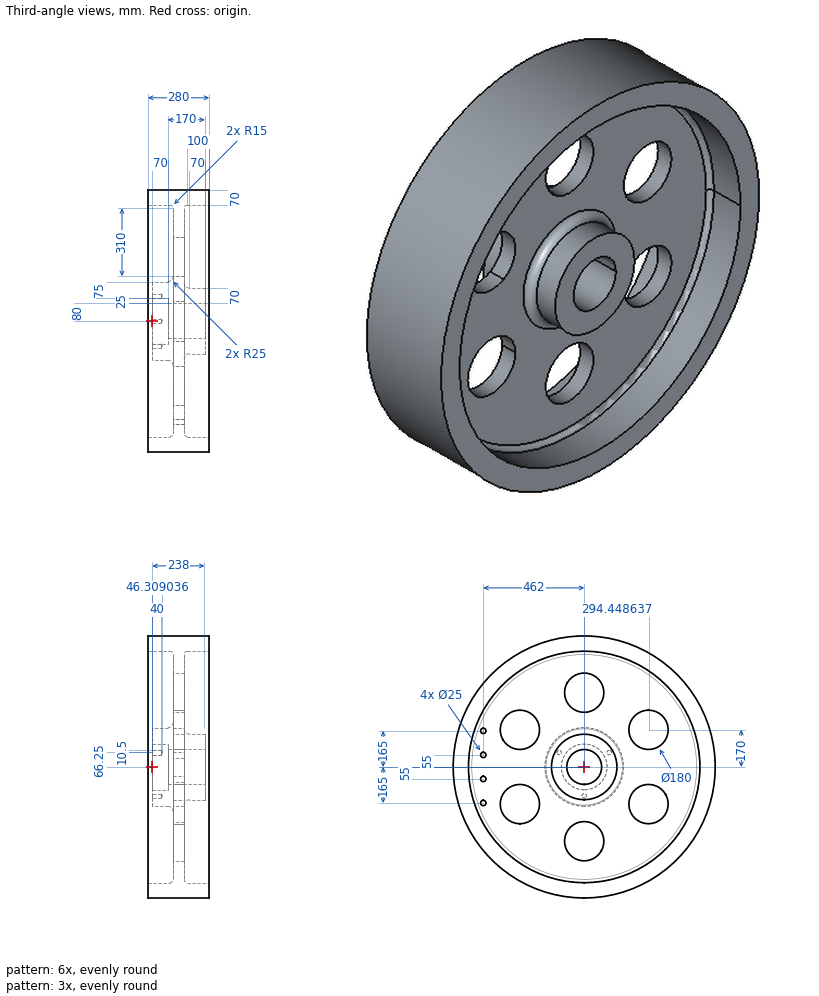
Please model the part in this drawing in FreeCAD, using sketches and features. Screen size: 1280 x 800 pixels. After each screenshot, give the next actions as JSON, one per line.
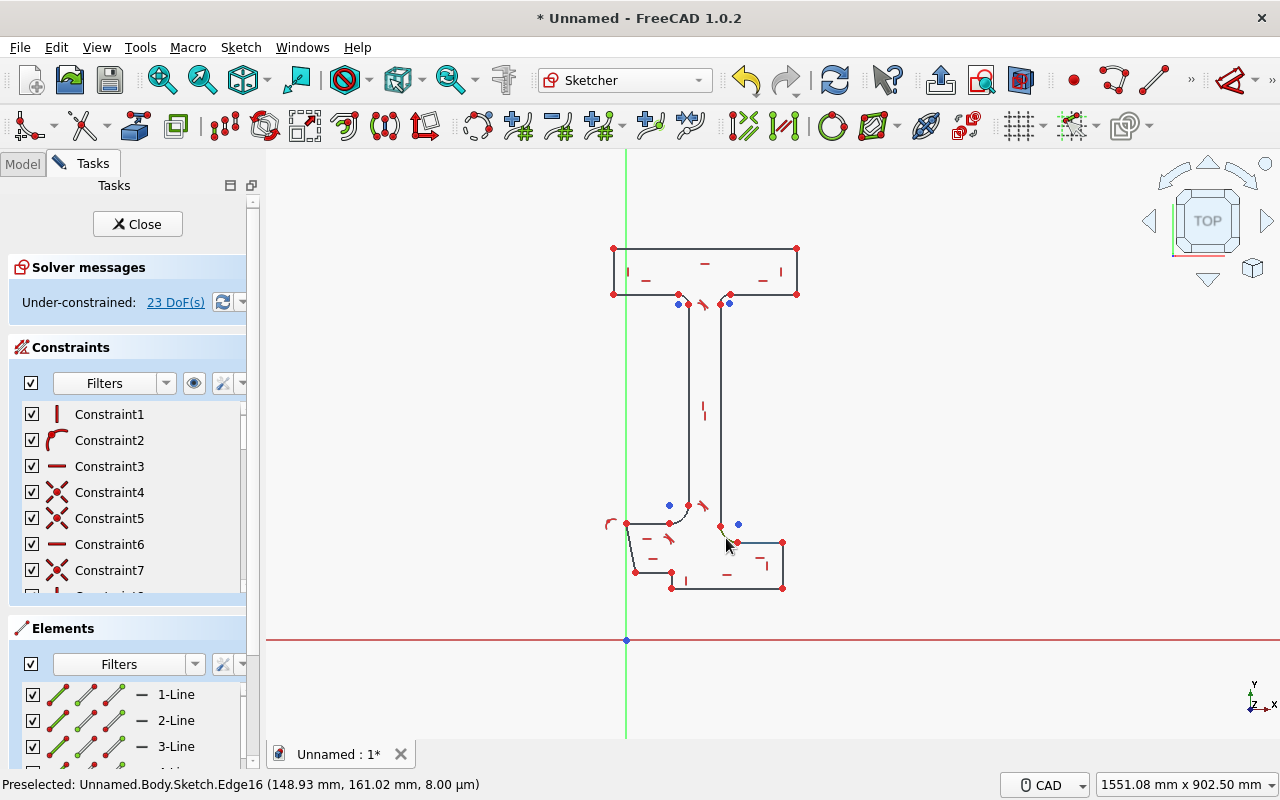
{"action": "key", "text": "t"}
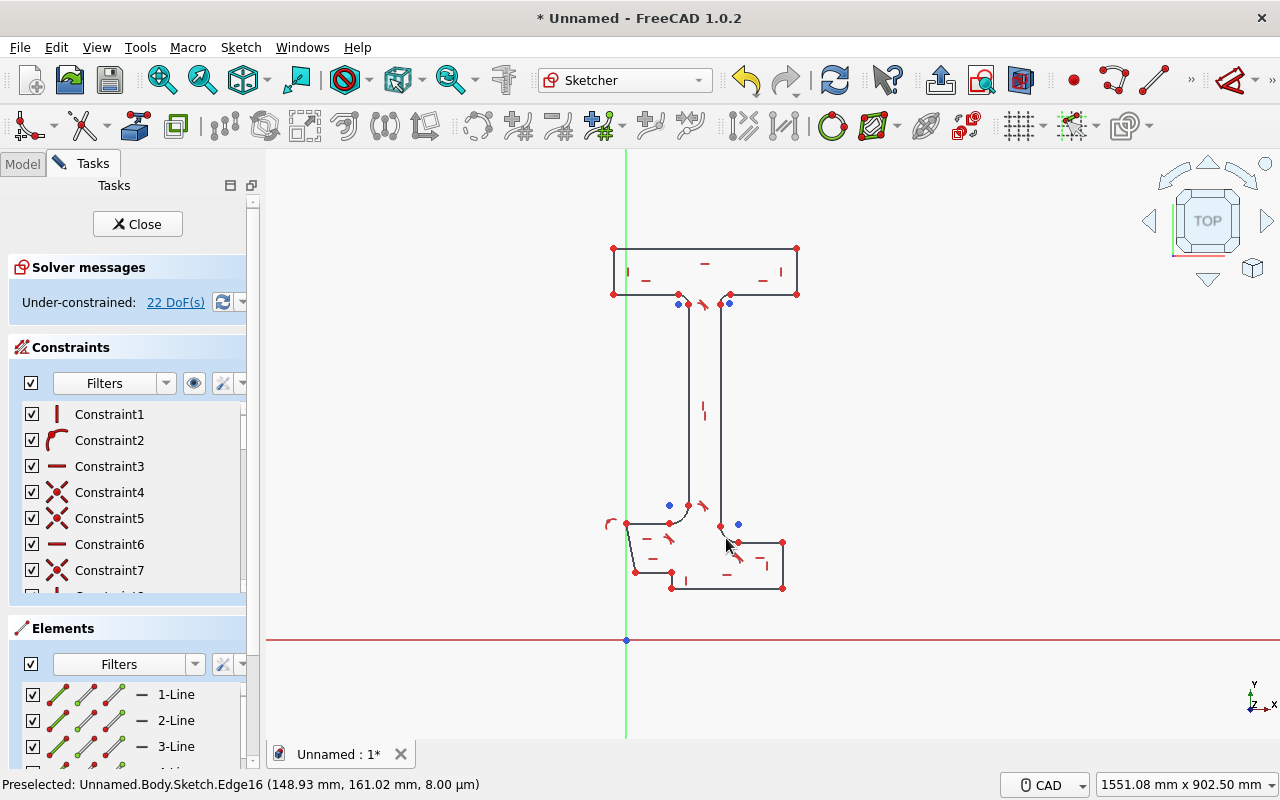
{"action": "left_click", "coordinate": [721, 460]}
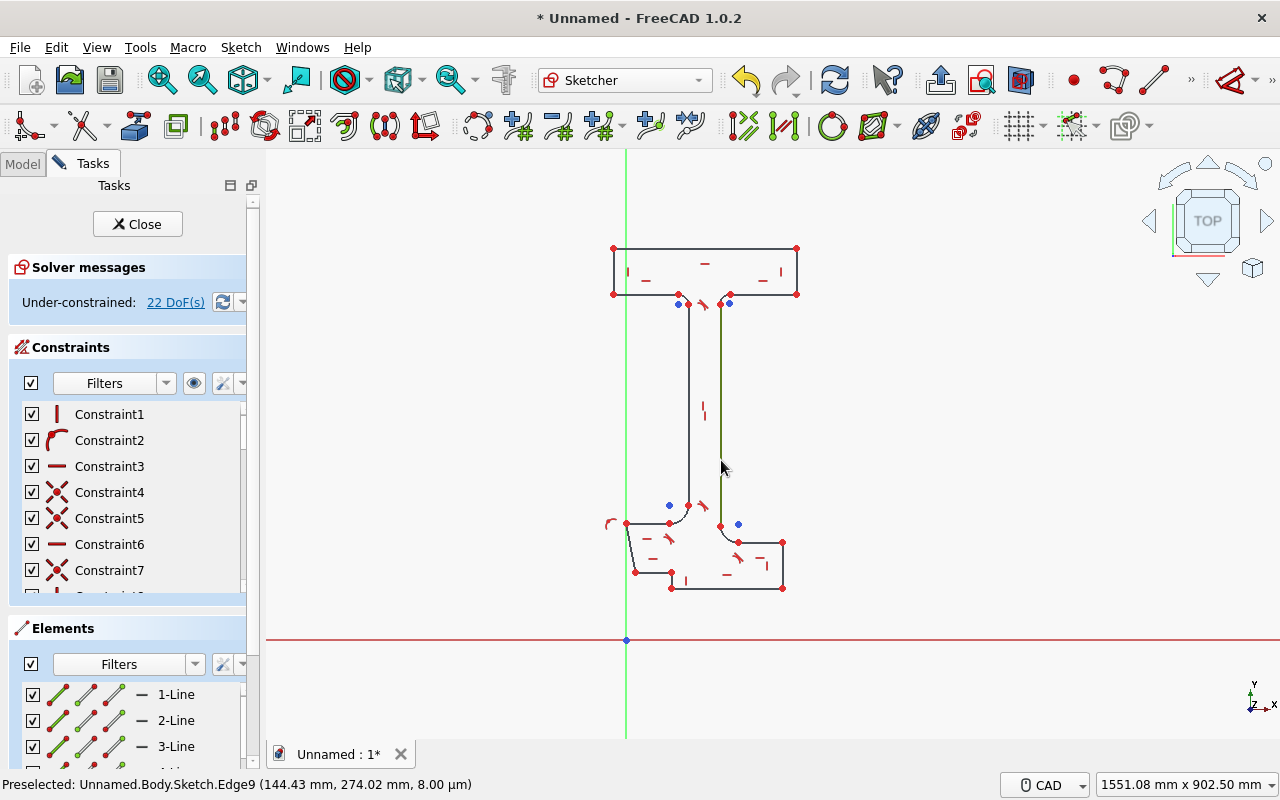
{"action": "left_click", "coordinate": [726, 538]}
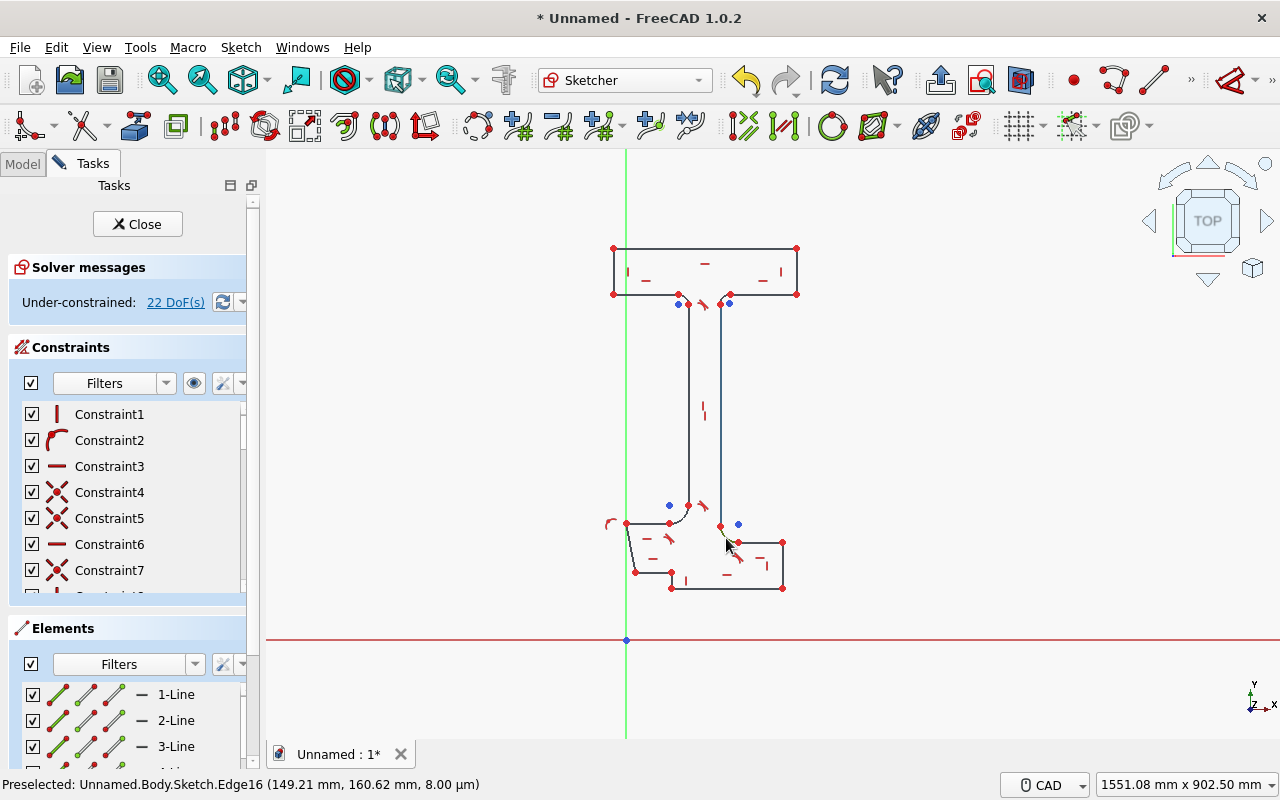
{"action": "key", "text": "t"}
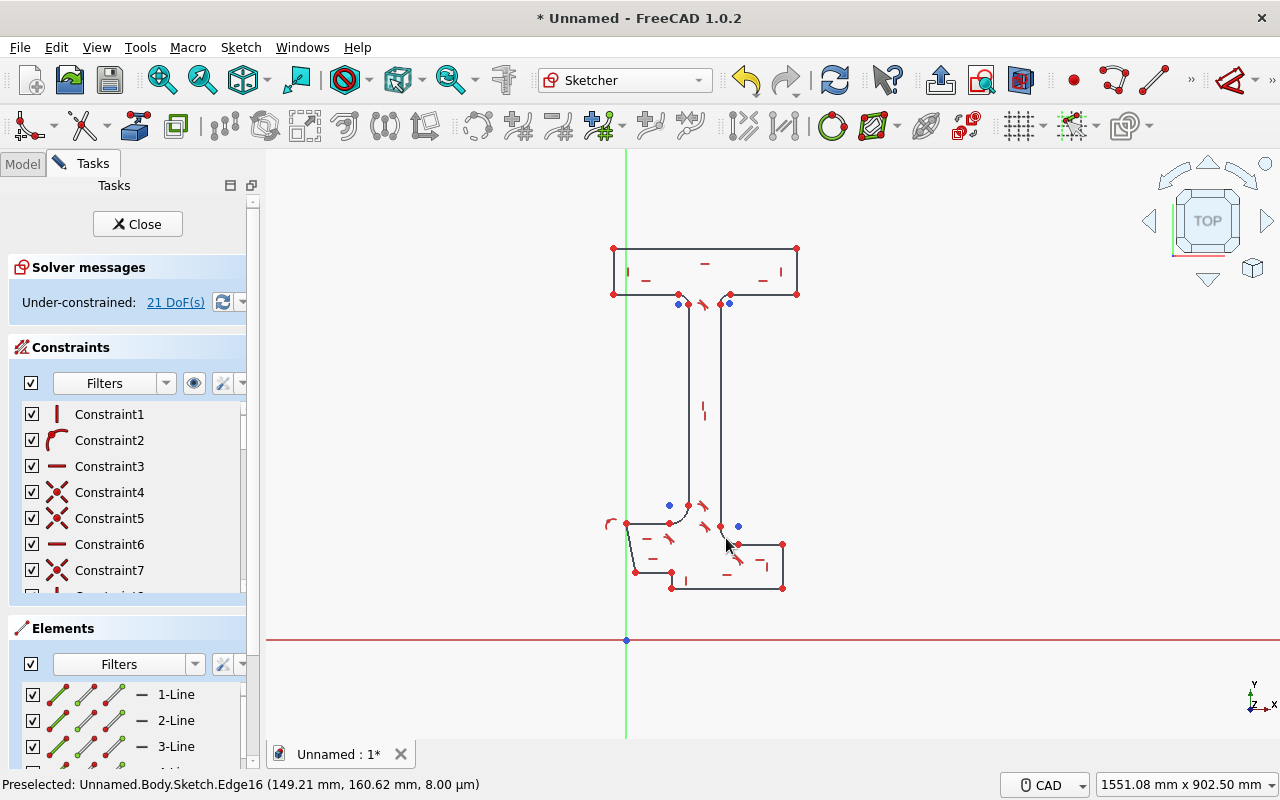
{"action": "left_click", "coordinate": [721, 460]}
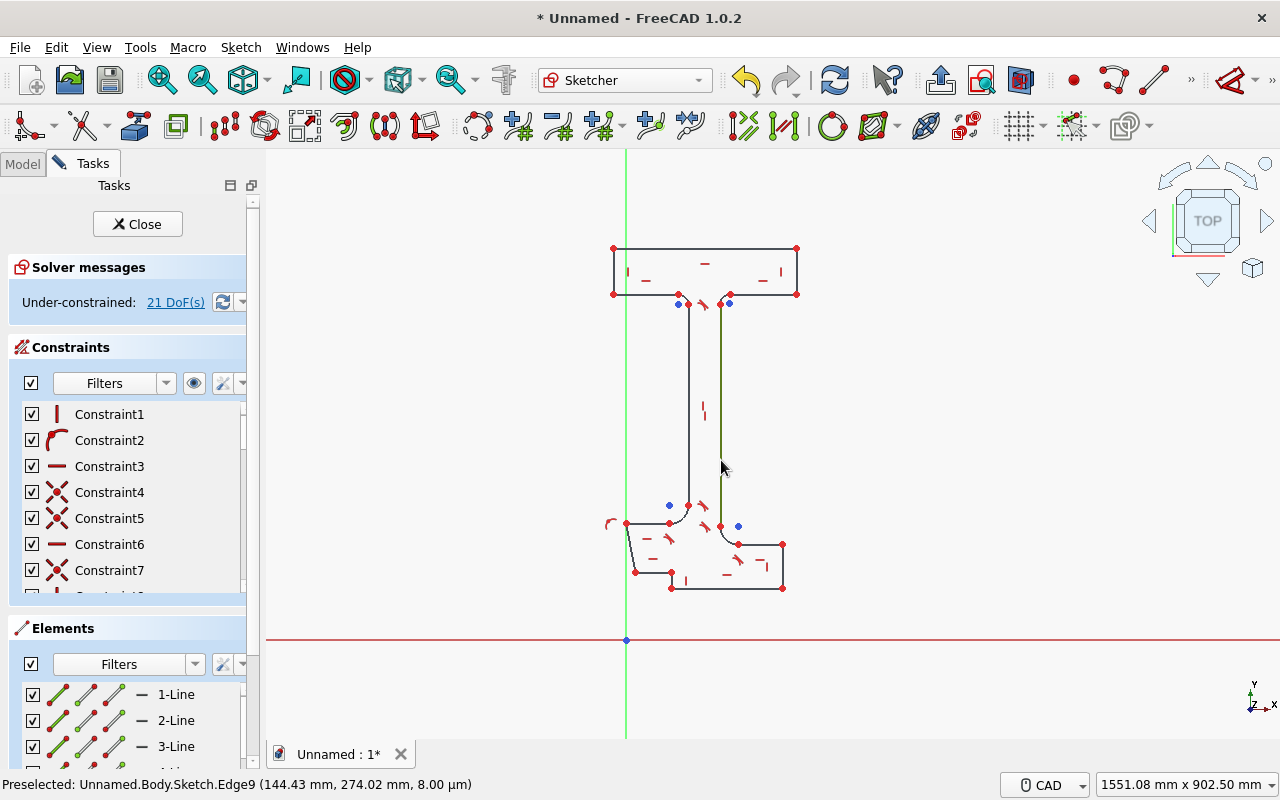
{"action": "scroll", "coordinate": [723, 297], "scroll_direction": "up", "scroll_amount": 3}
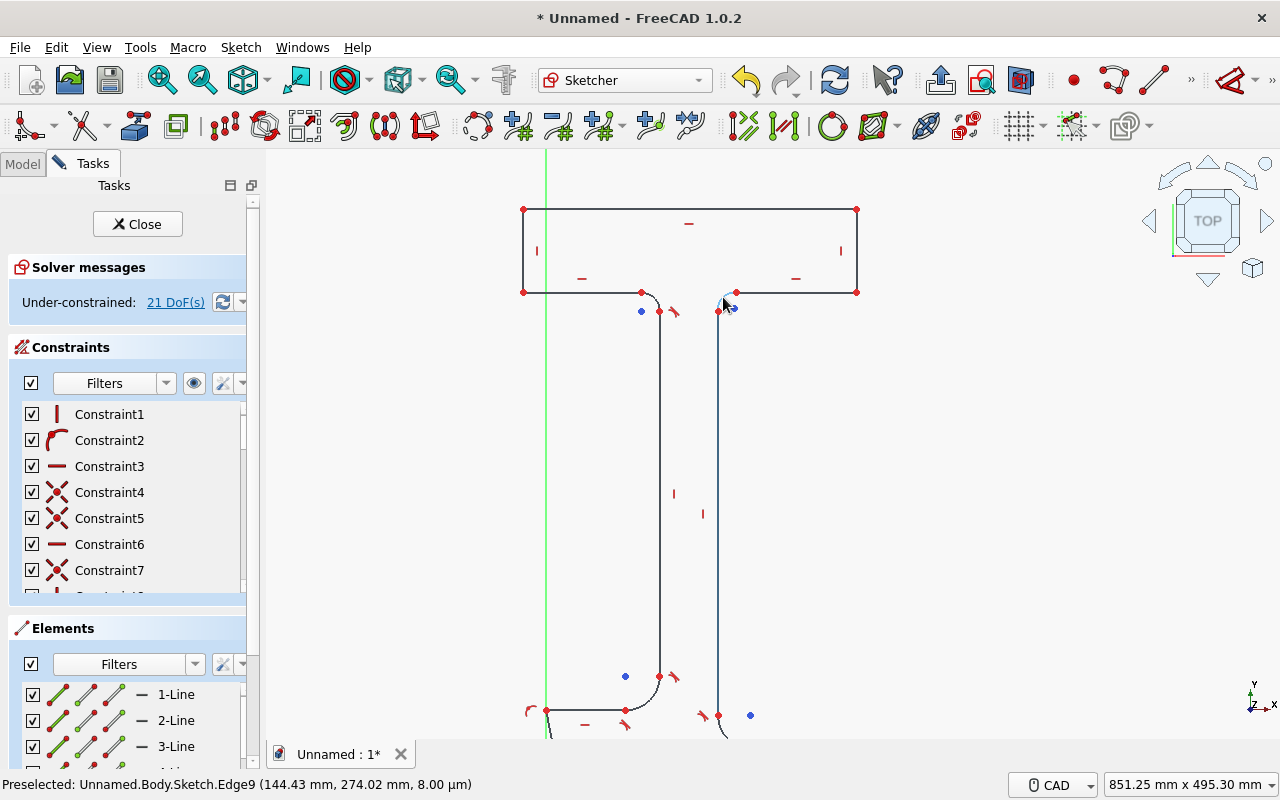
{"action": "left_click", "coordinate": [723, 297]}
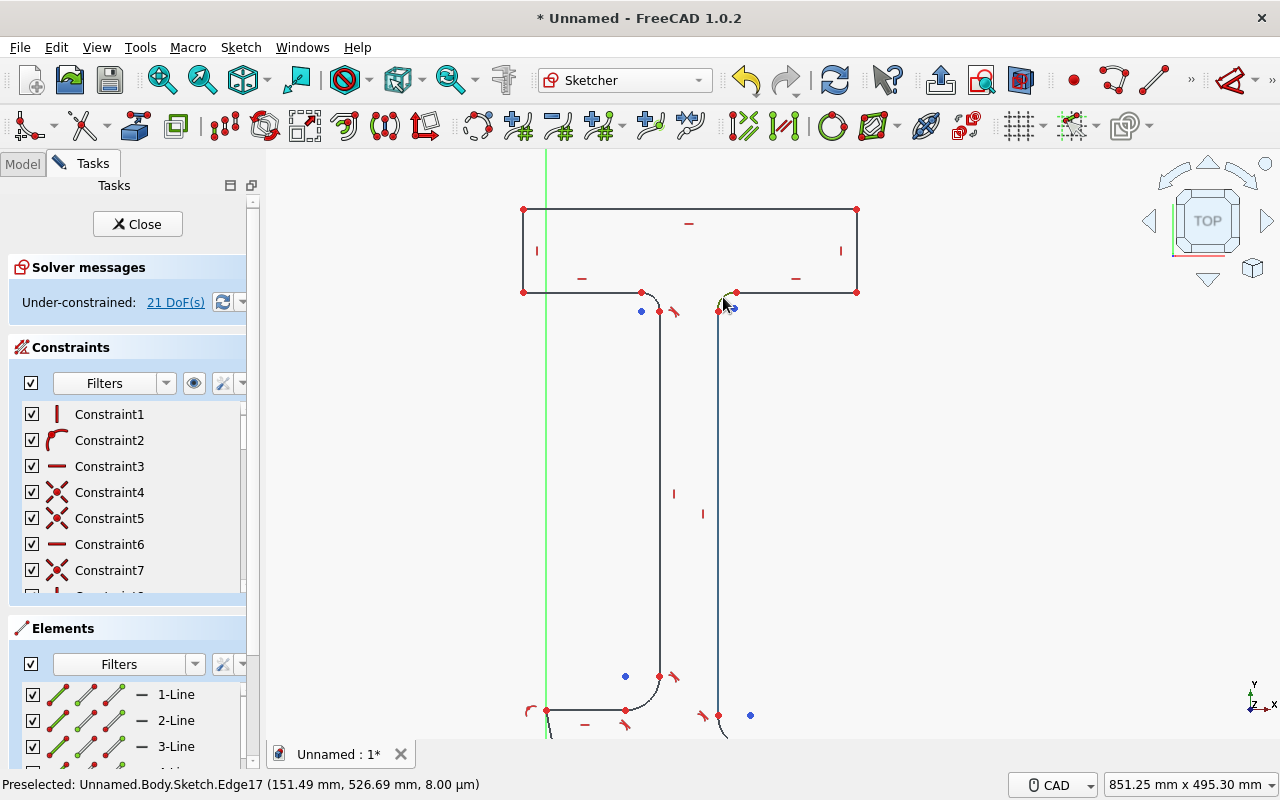
{"action": "key", "text": "t"}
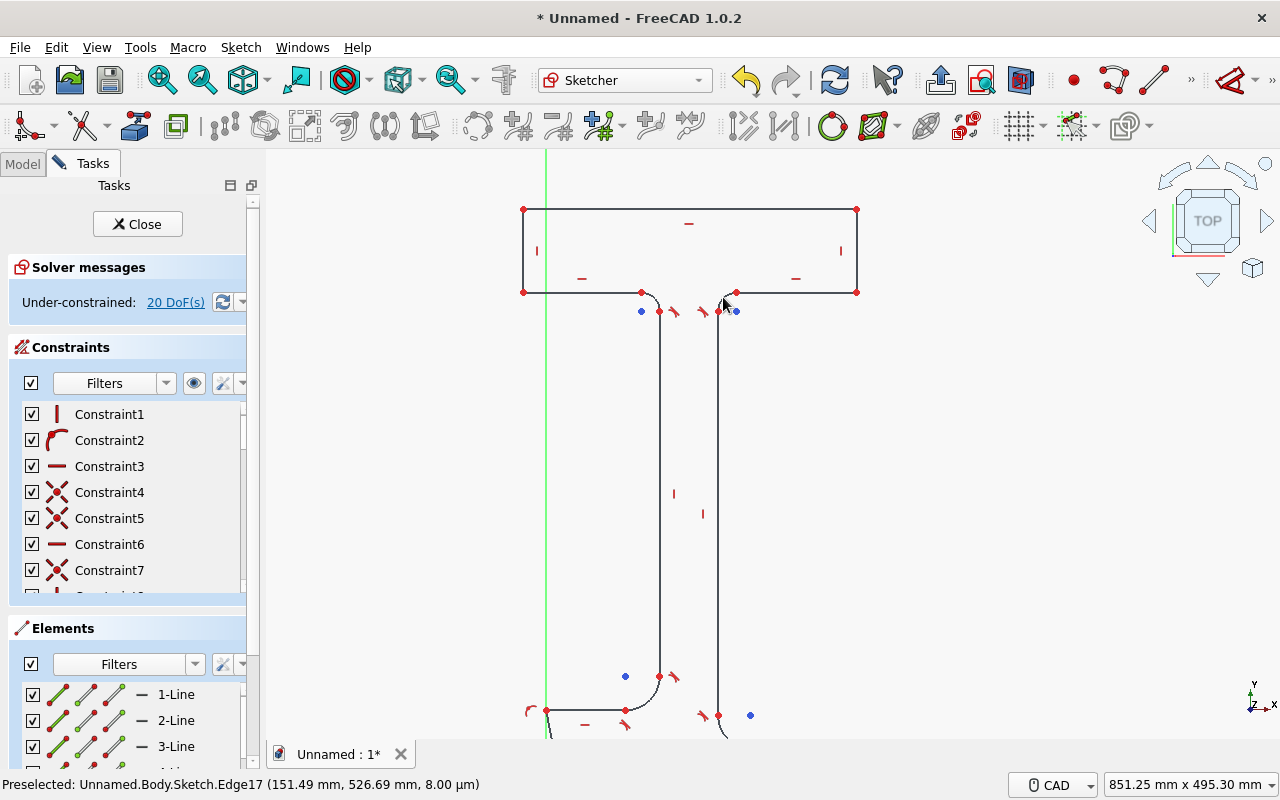
{"action": "left_click", "coordinate": [772, 293]}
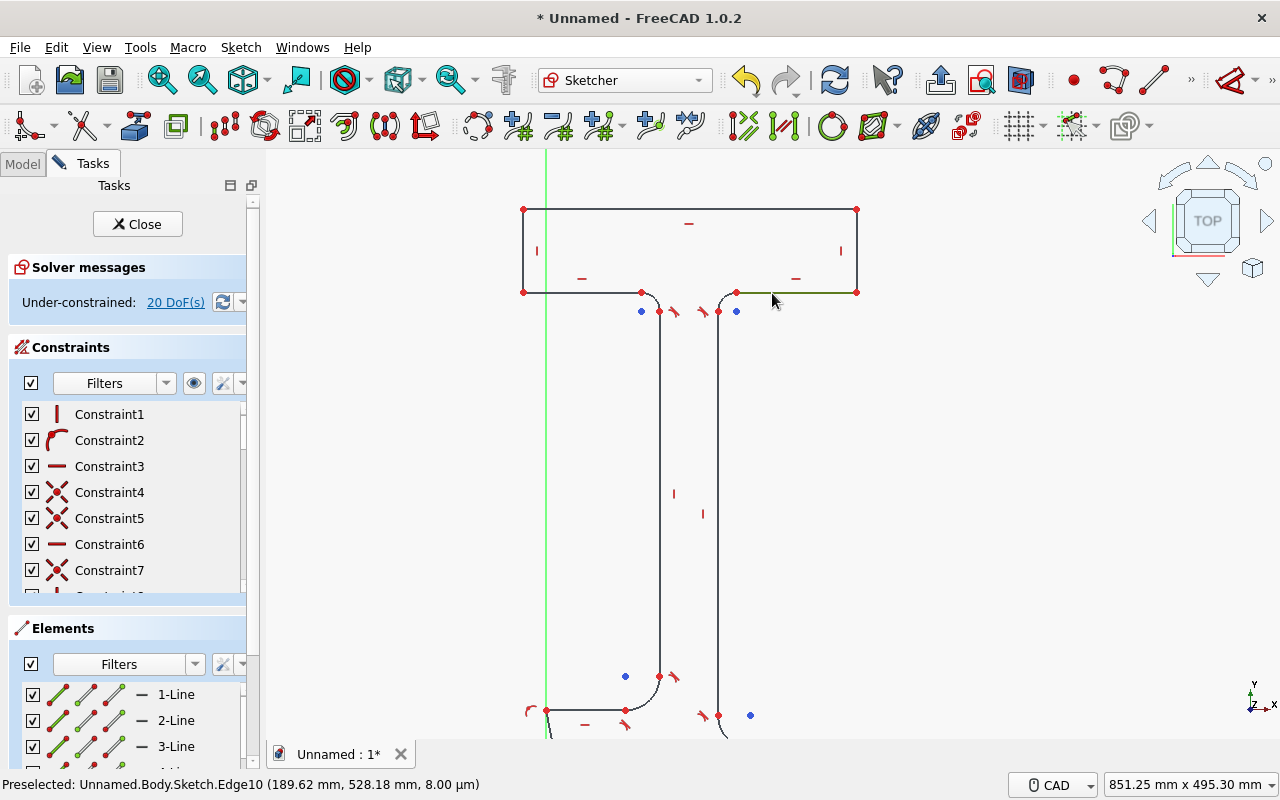
{"action": "left_click", "coordinate": [723, 298]}